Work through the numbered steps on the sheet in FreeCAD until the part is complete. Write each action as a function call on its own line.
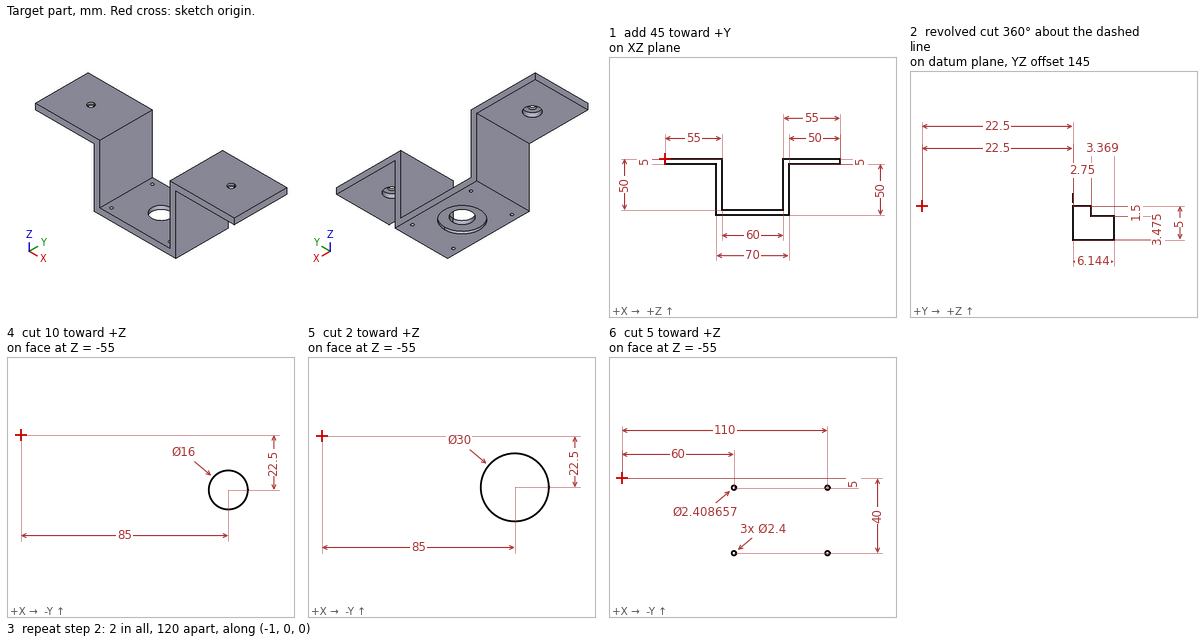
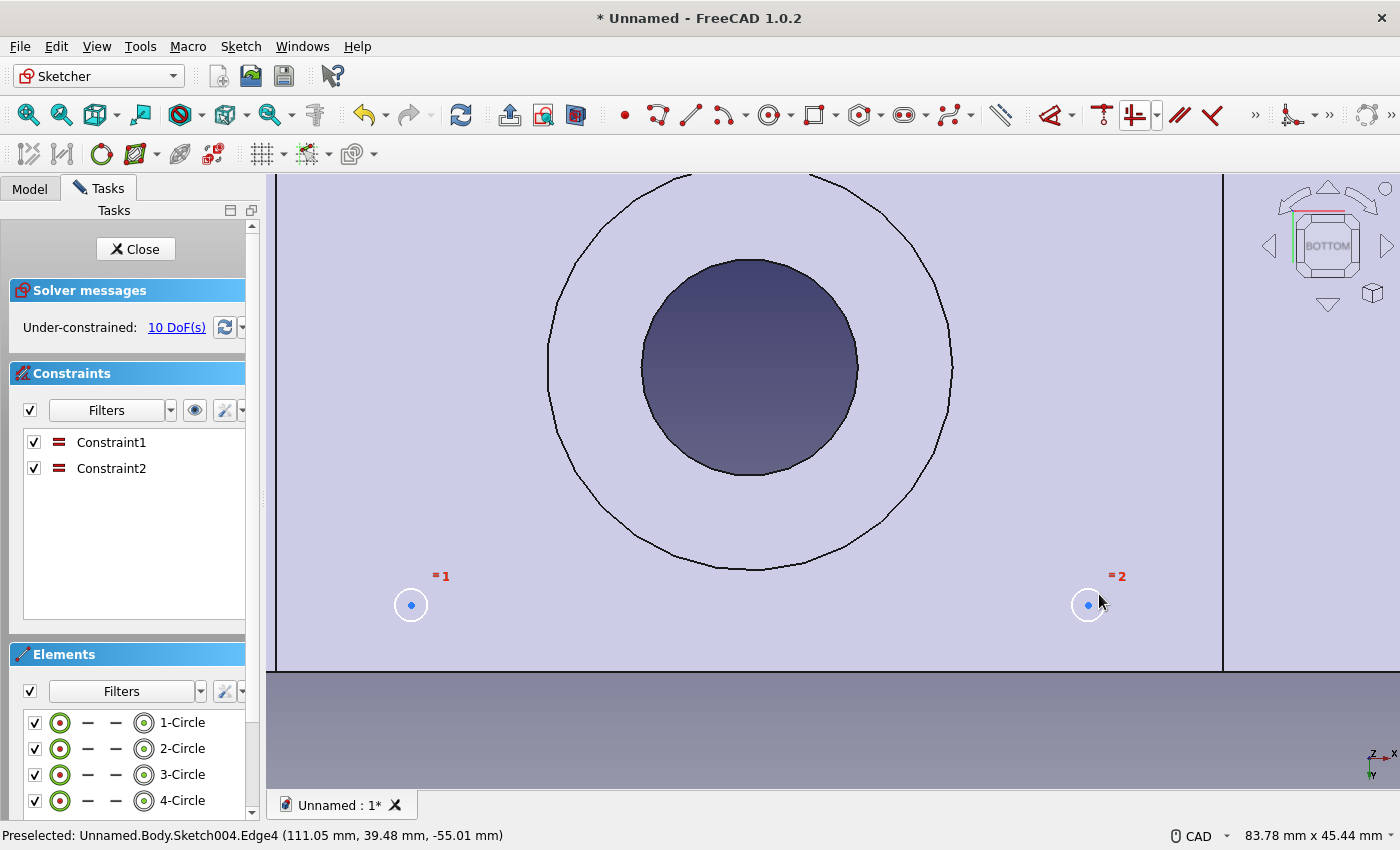
scroll(1101, 595, down, 4)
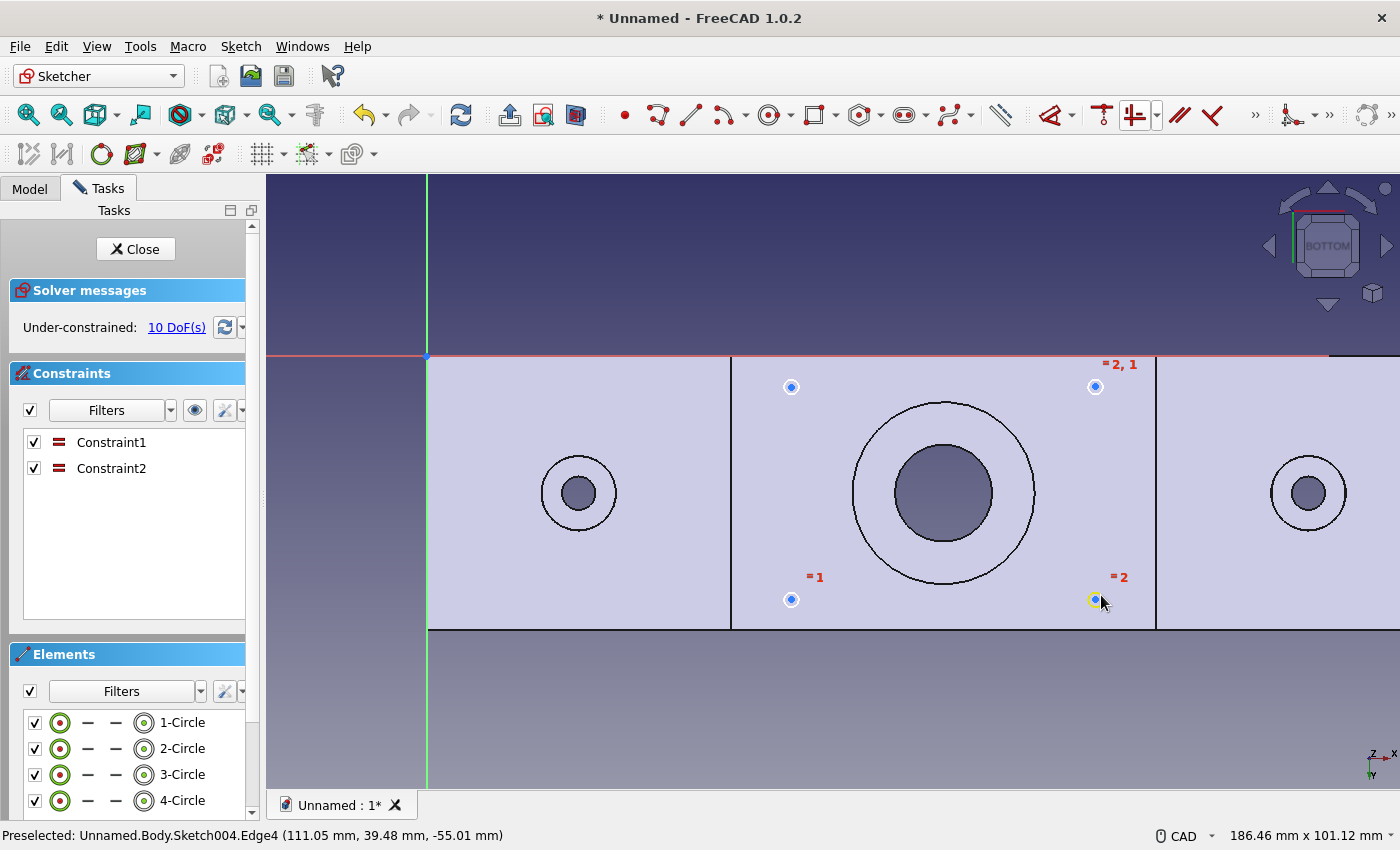
click(791, 387)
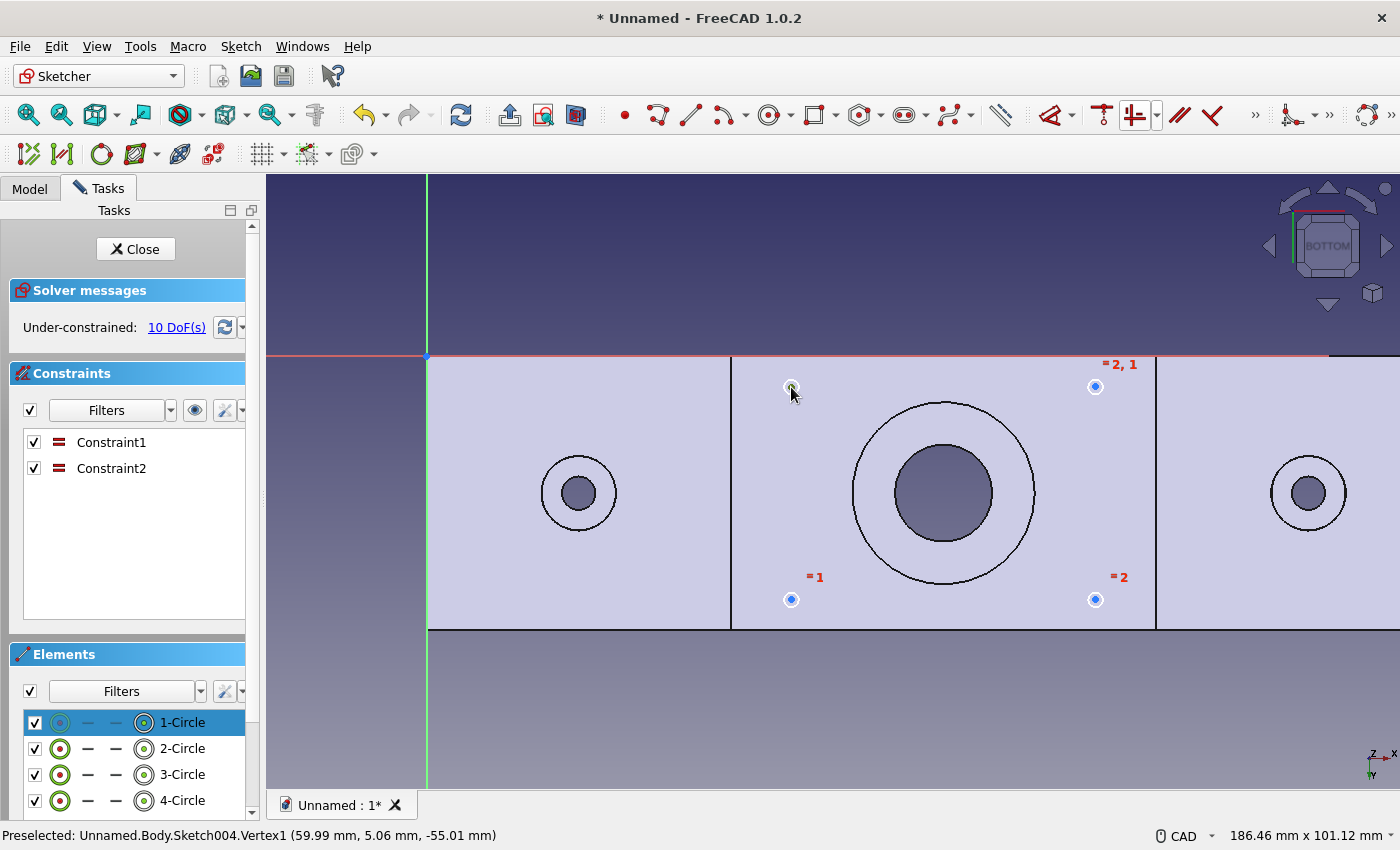
click(791, 600)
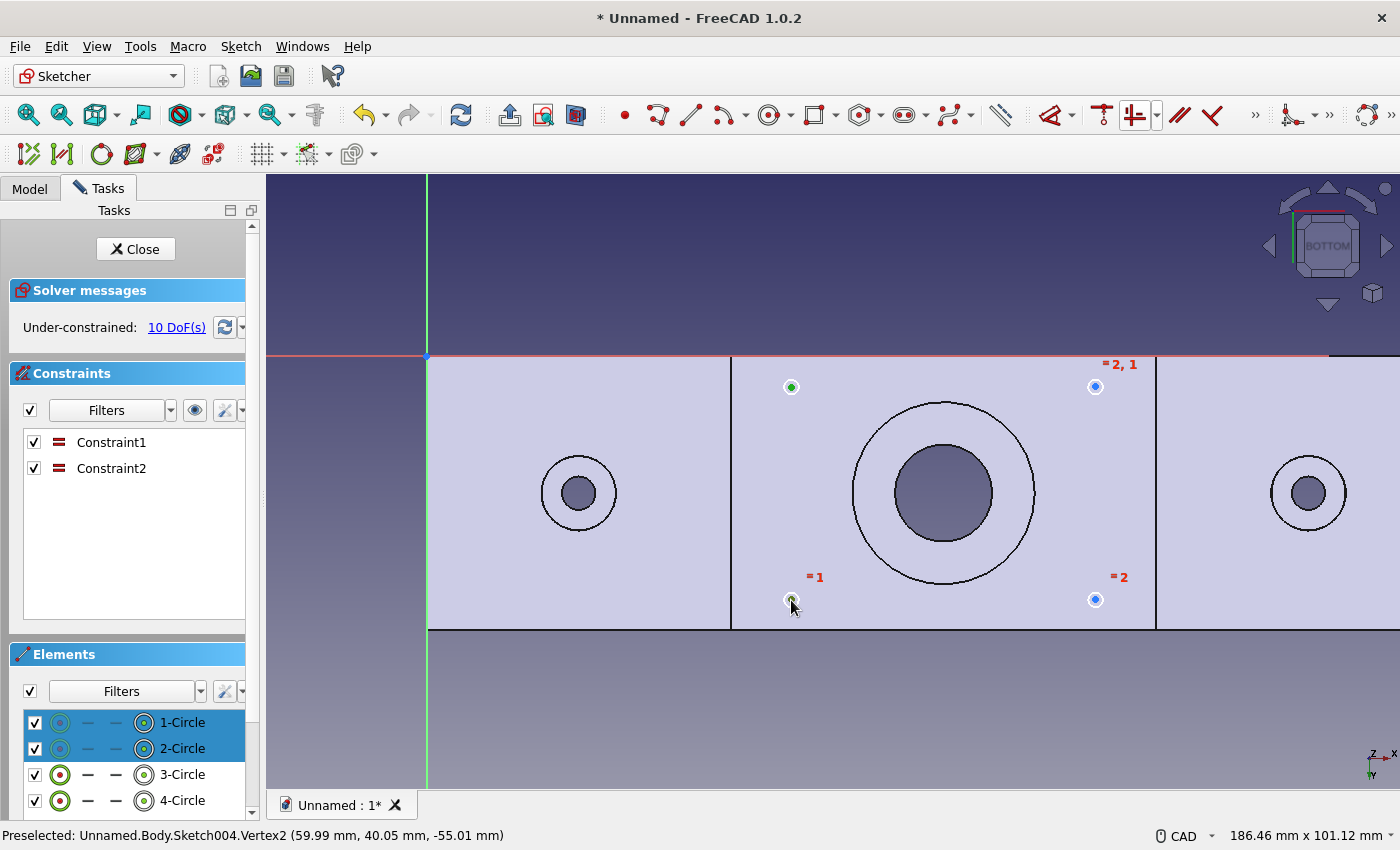
key(v)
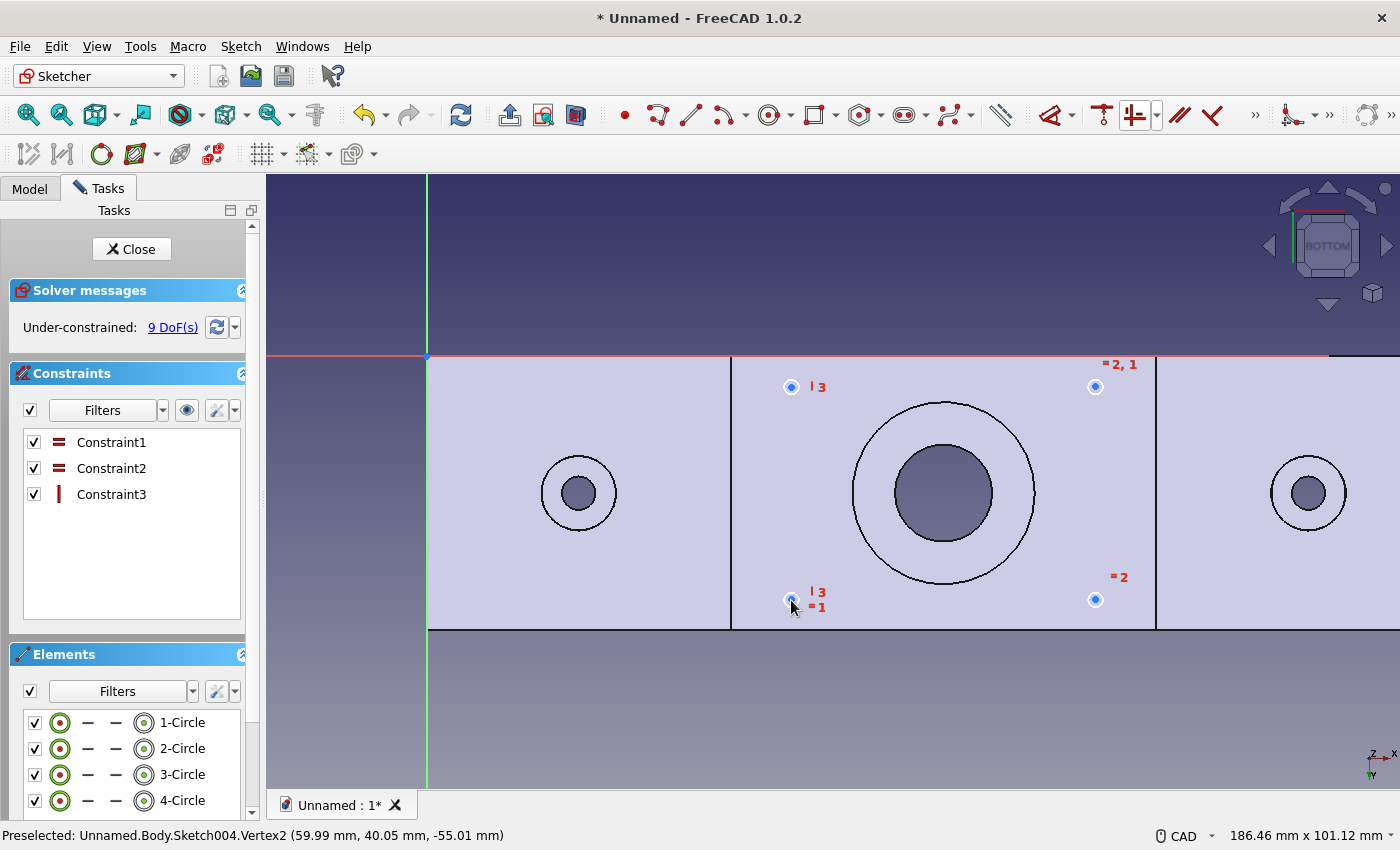
click(791, 387)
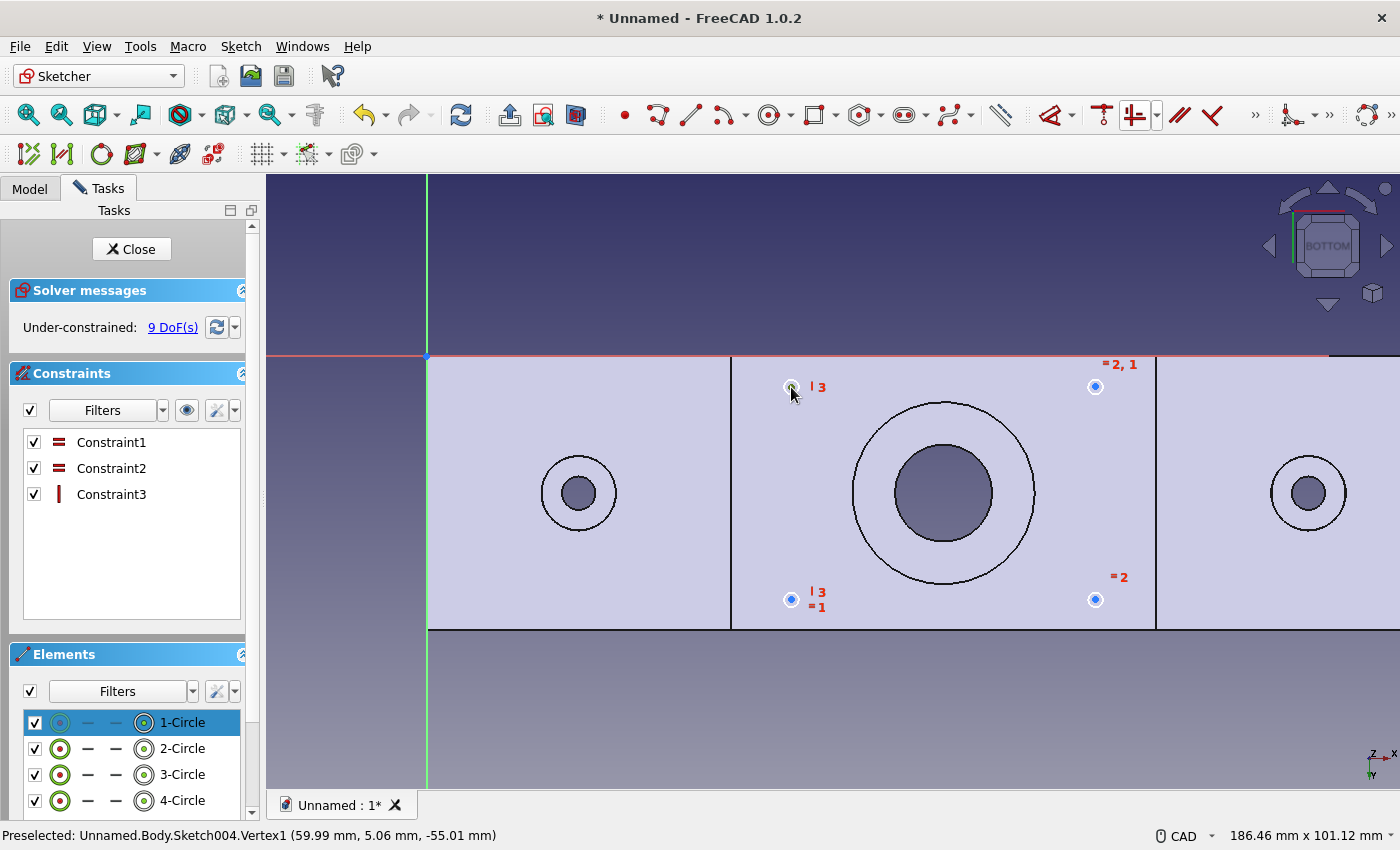
click(1096, 387)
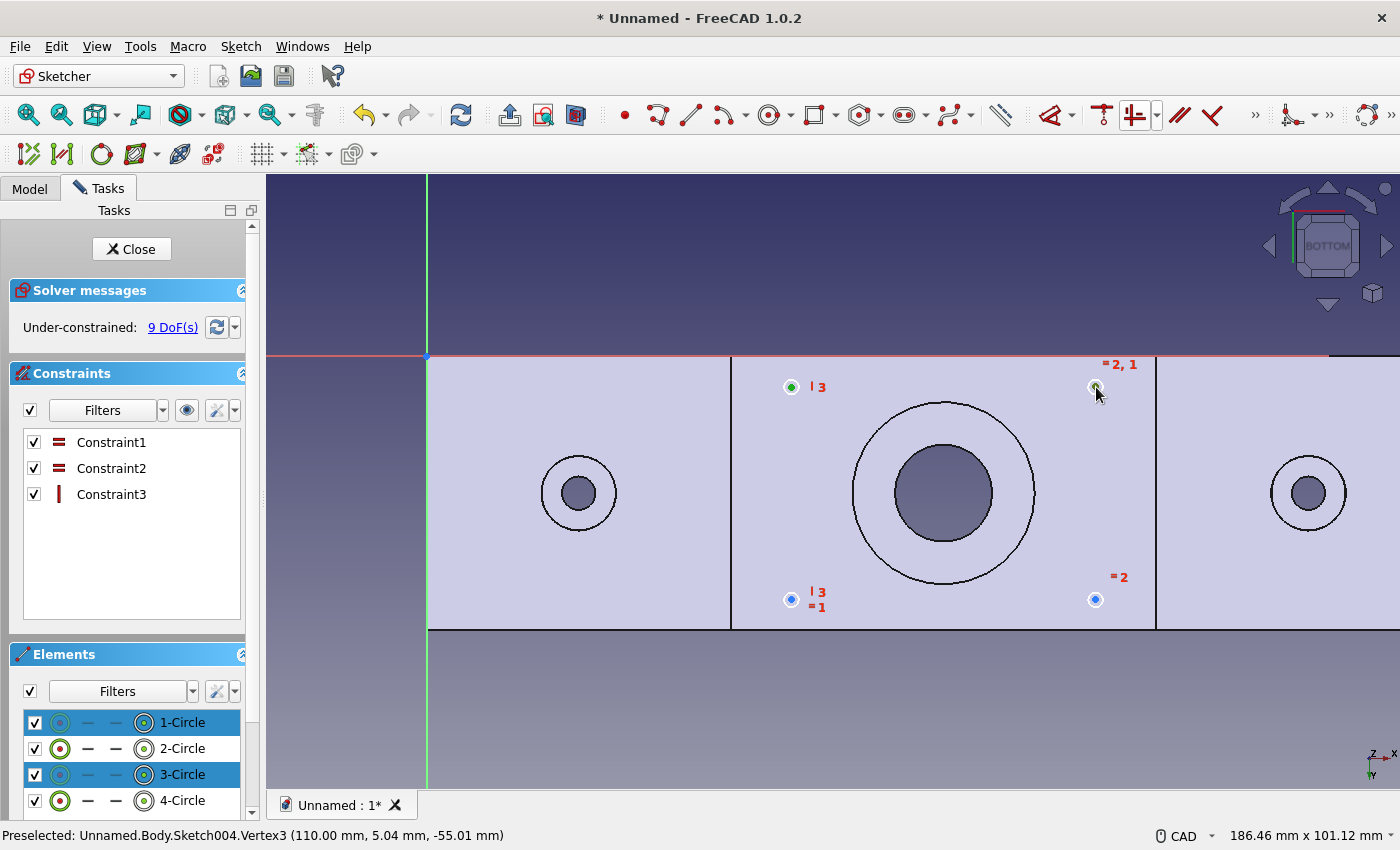
key(h)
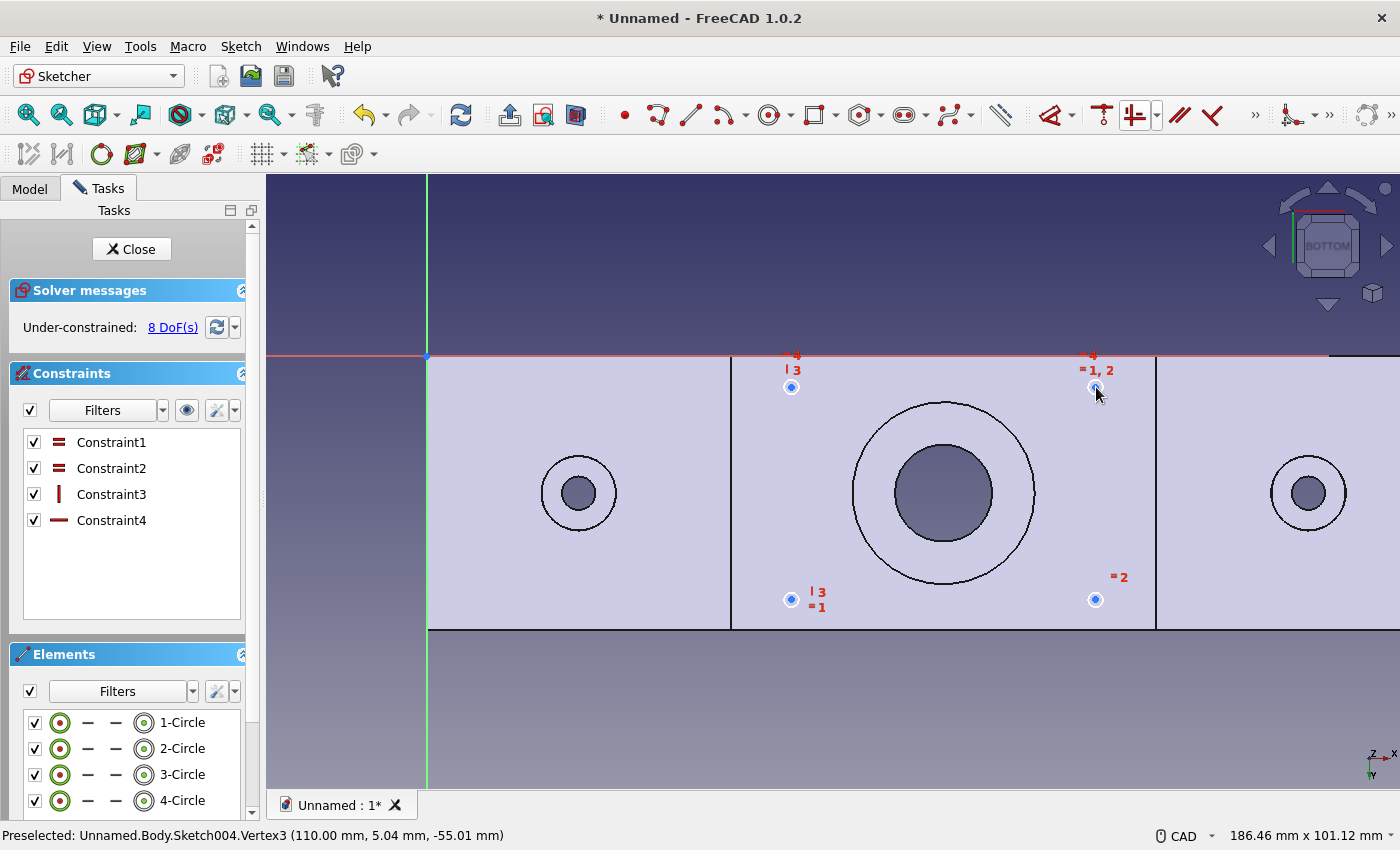
click(1096, 387)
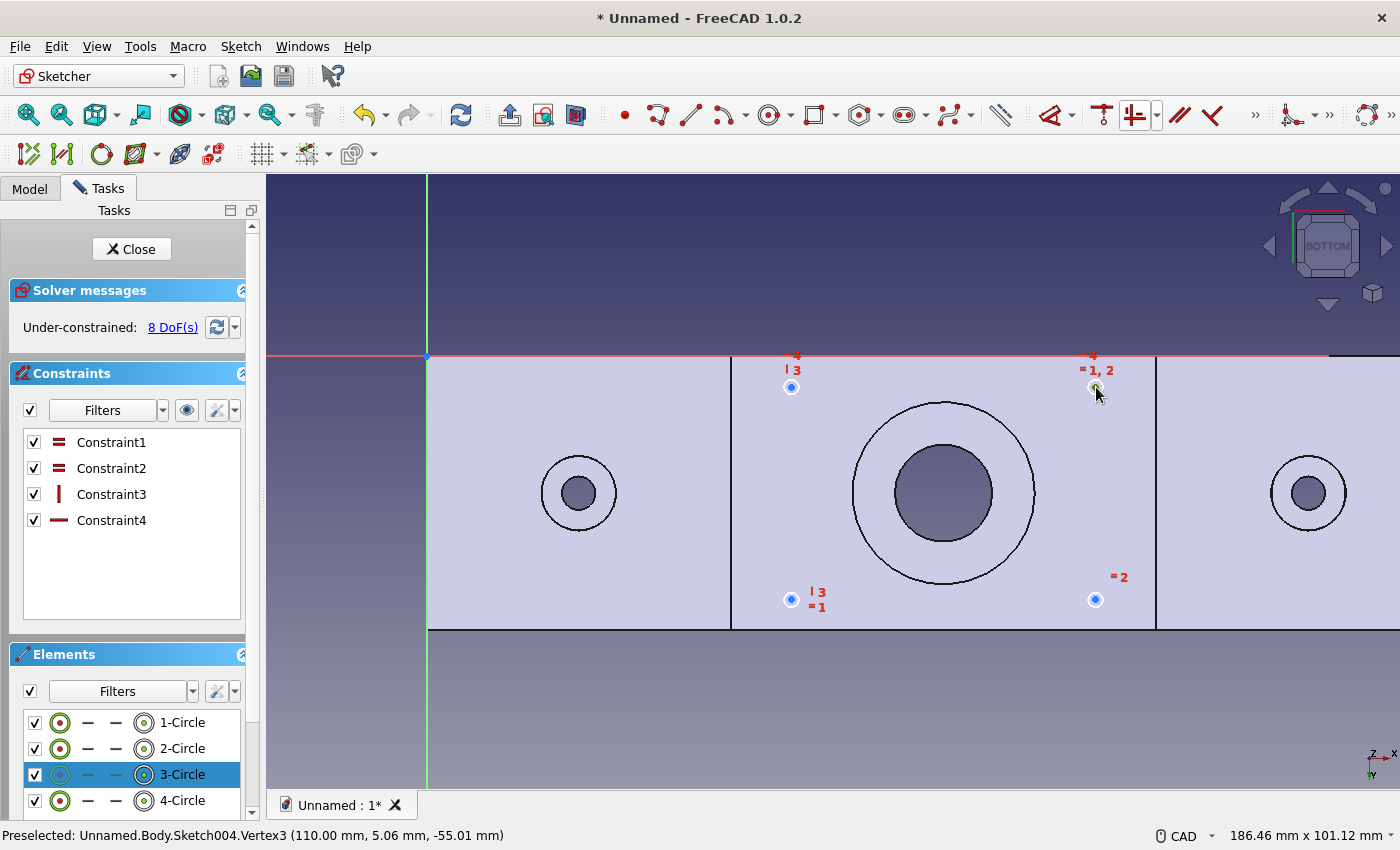
click(1096, 600)